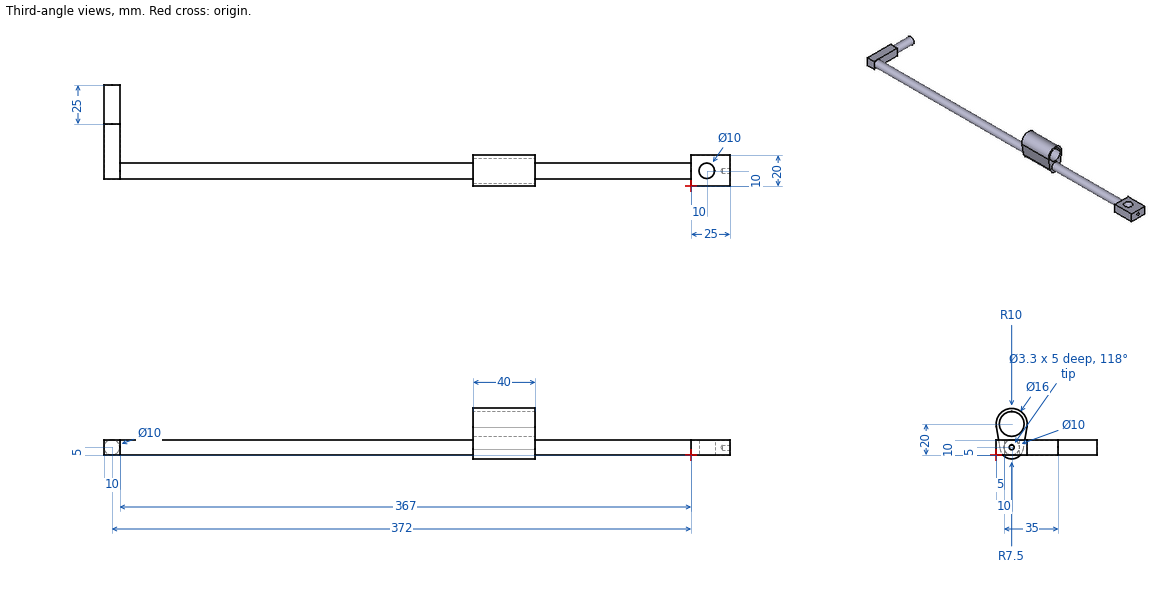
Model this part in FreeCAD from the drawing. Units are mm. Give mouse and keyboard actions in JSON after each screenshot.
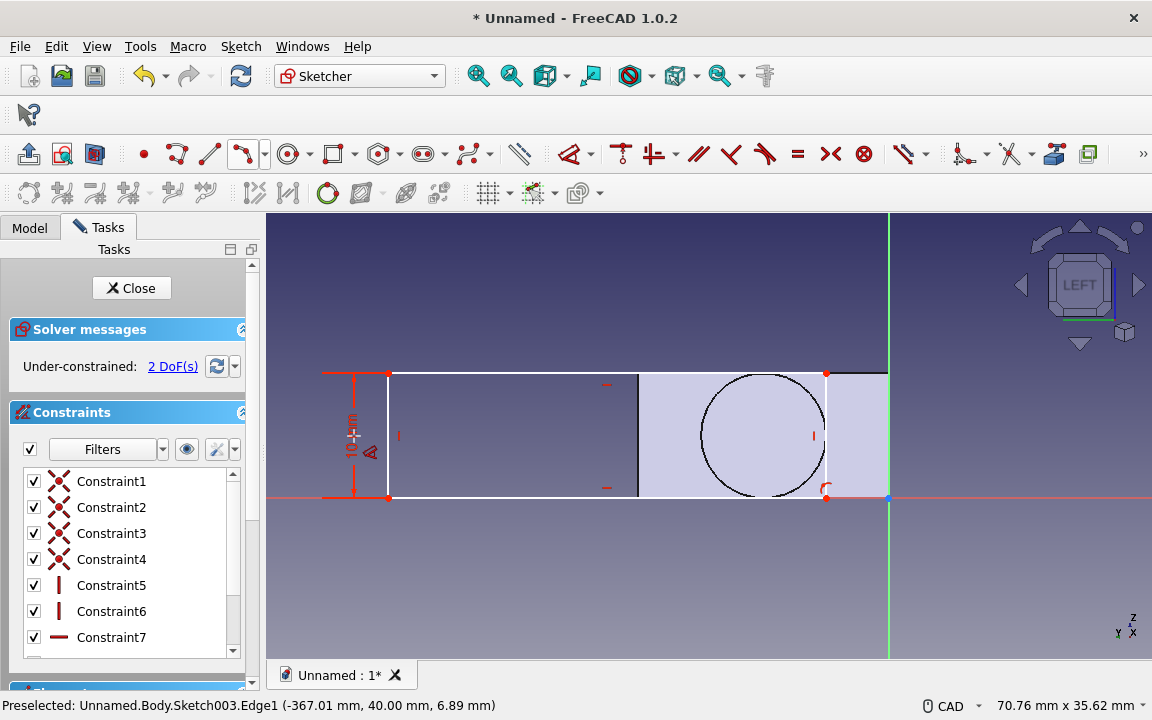
{"action": "left_click", "coordinate": [519, 498]}
{"action": "left_click", "coordinate": [607, 532]}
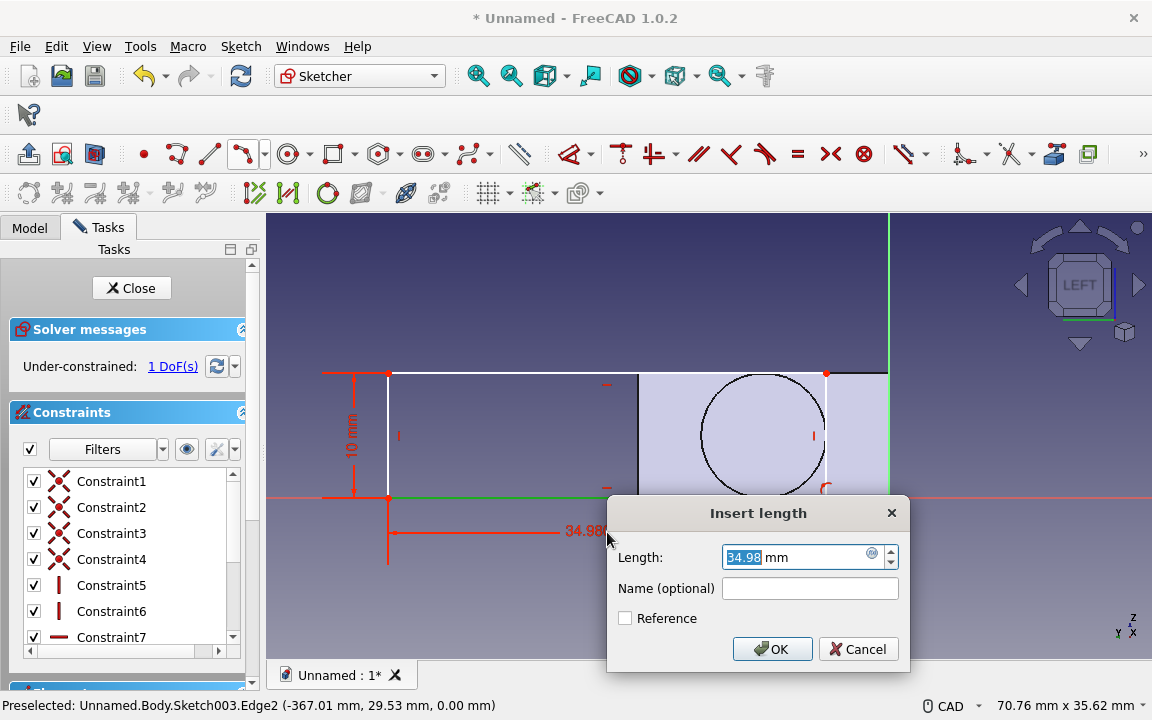
{"action": "type", "text": "35"}
{"action": "key", "text": "Return"}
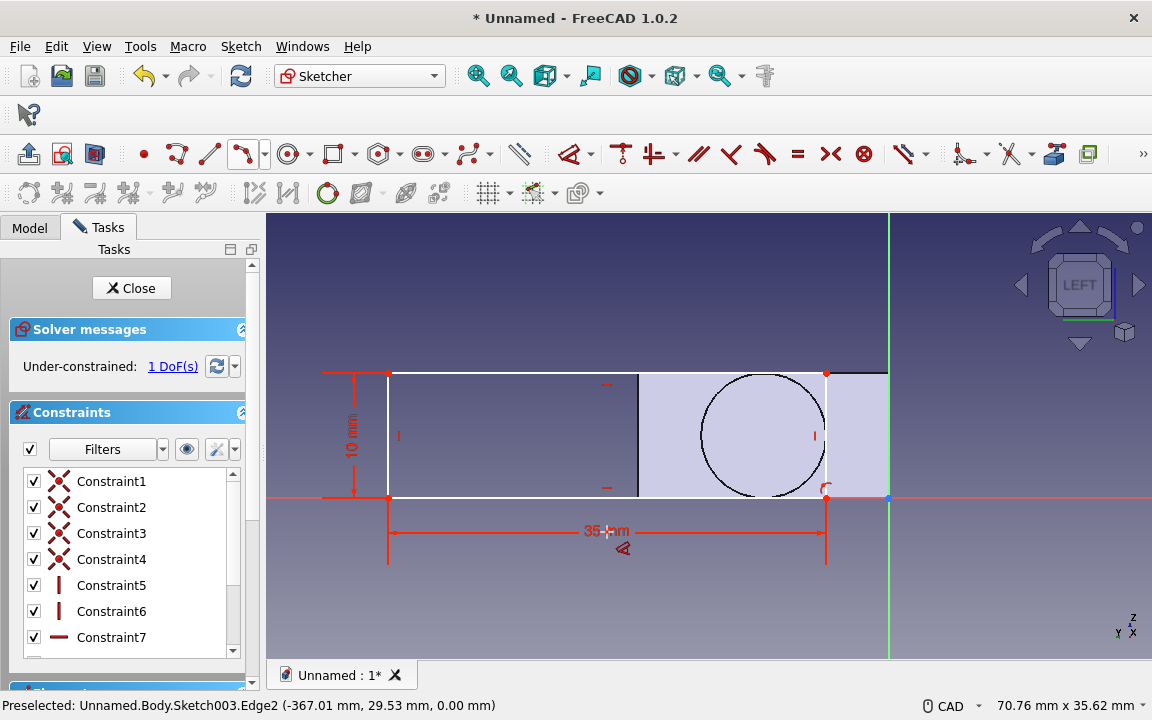
{"action": "left_click", "coordinate": [826, 498]}
{"action": "left_click", "coordinate": [858, 532]}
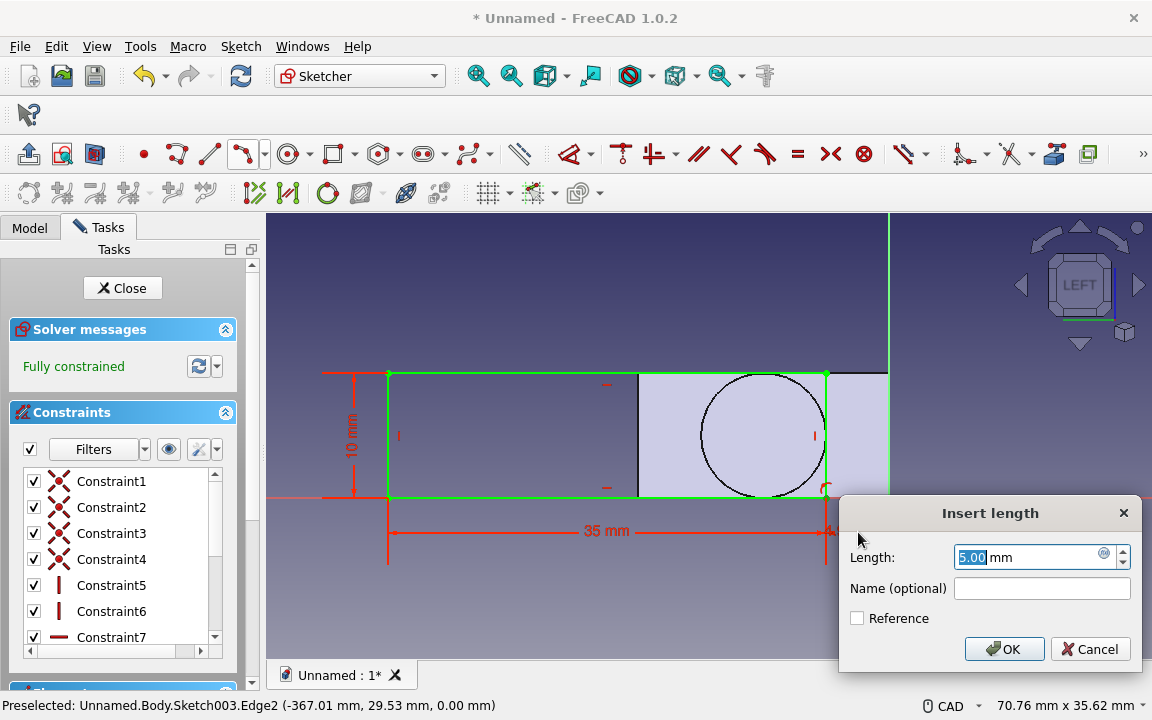
{"action": "type", "text": "5"}
{"action": "key", "text": "Return"}
{"action": "key", "text": "Escape"}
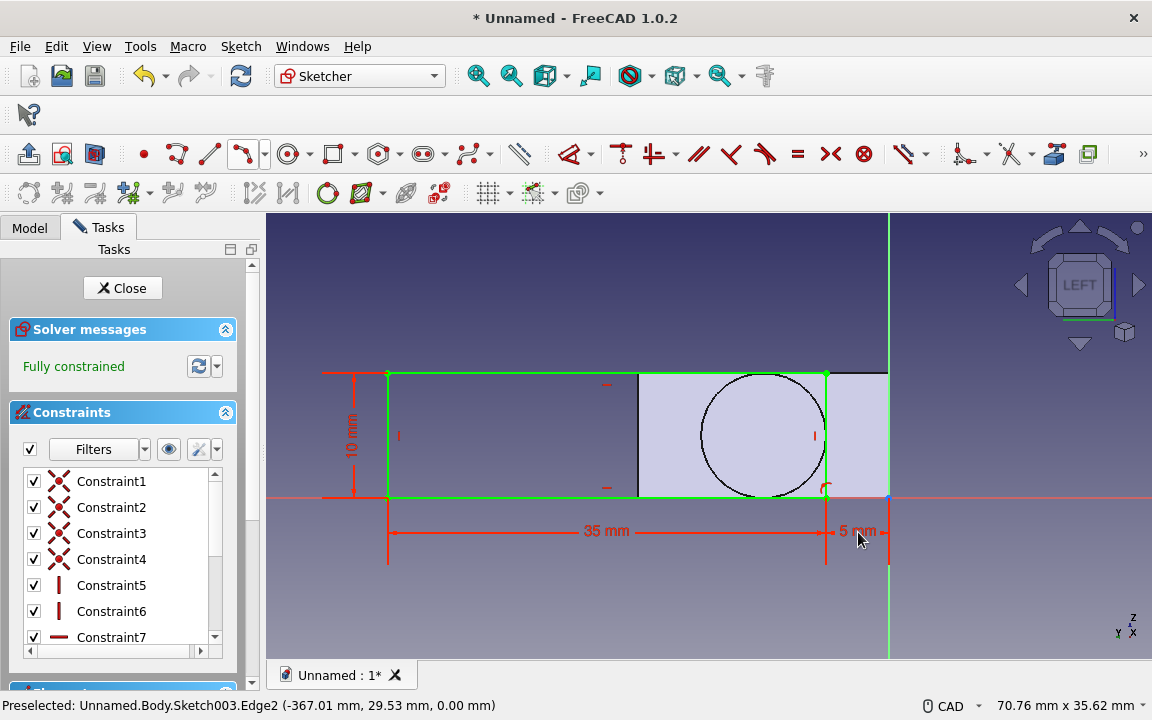
{"action": "left_click", "coordinate": [123, 288]}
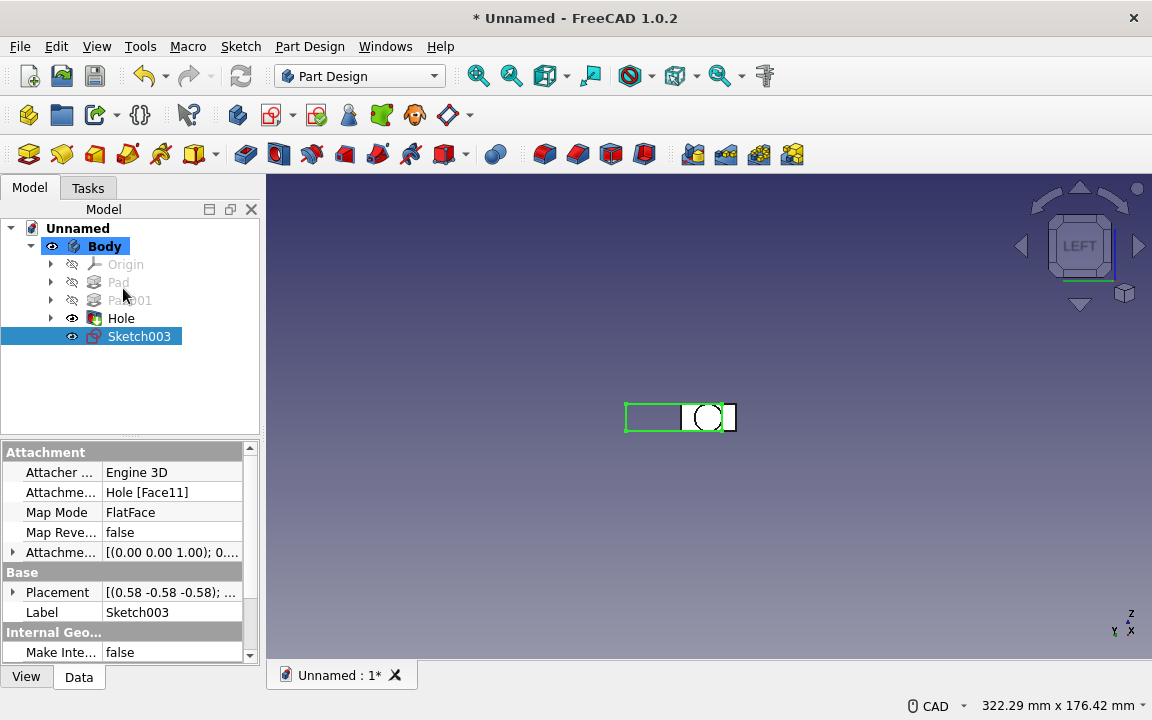
{"action": "left_click", "coordinate": [29, 154]}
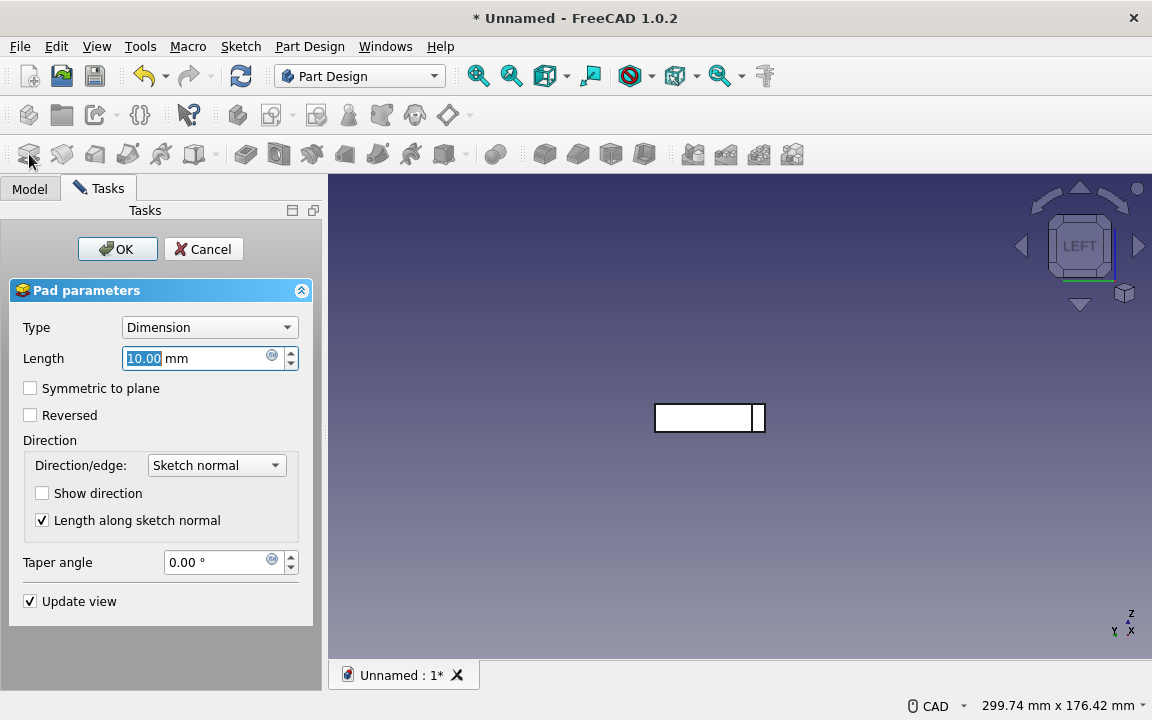
{"action": "type", "text": "10"}
{"action": "key", "text": "Tab"}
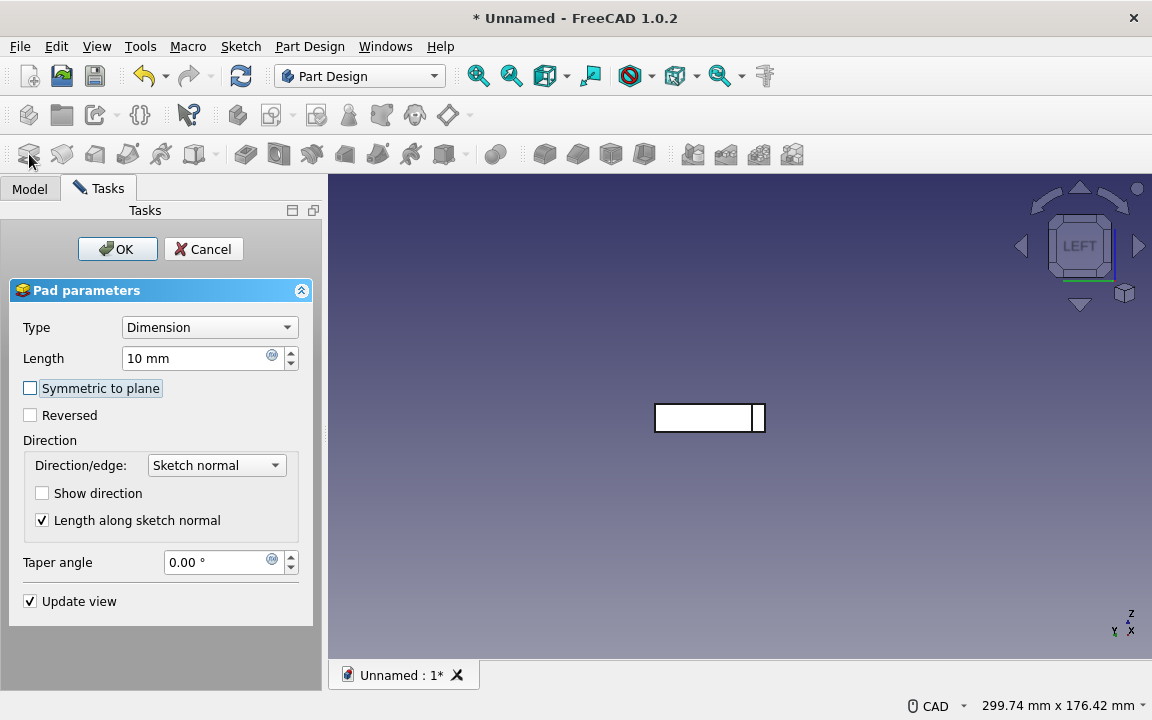
{"action": "left_click", "coordinate": [118, 249]}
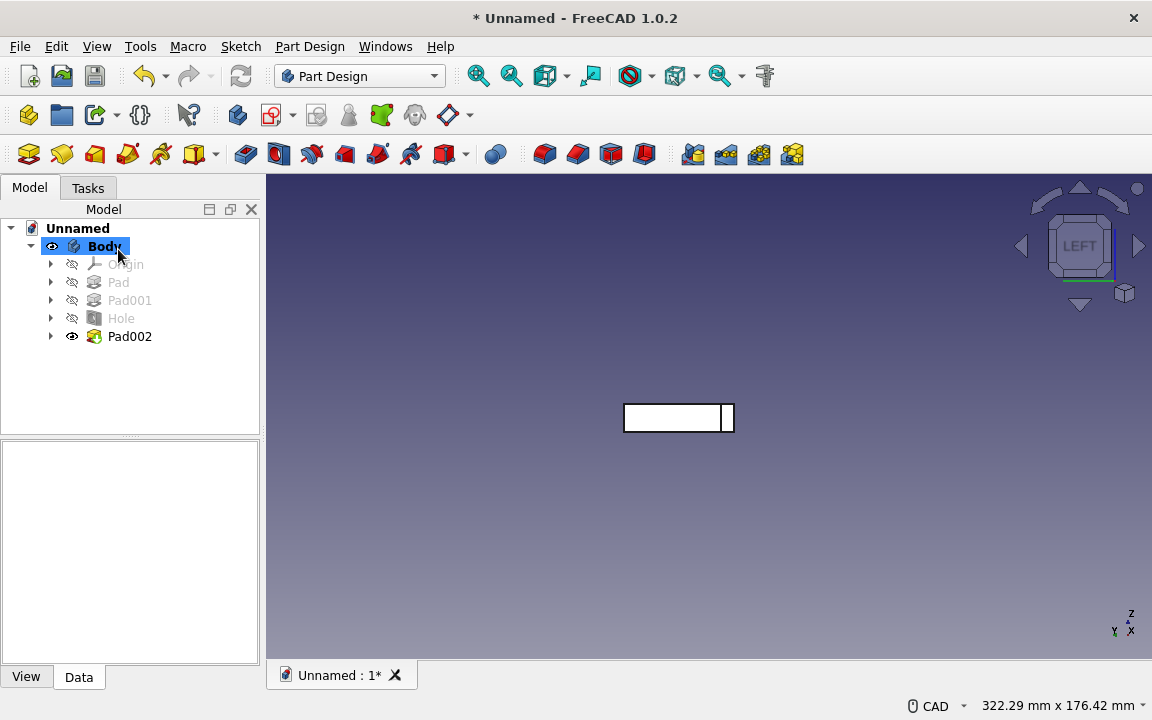
{"action": "key", "text": "v f"}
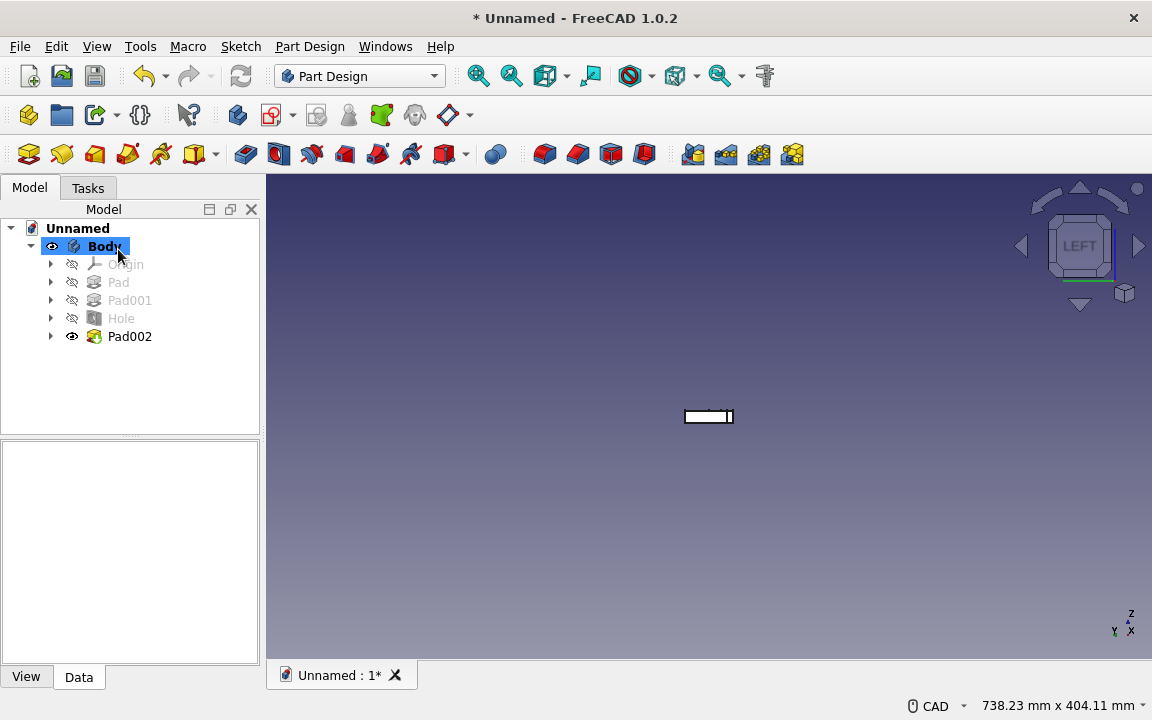
{"action": "key", "text": "4"}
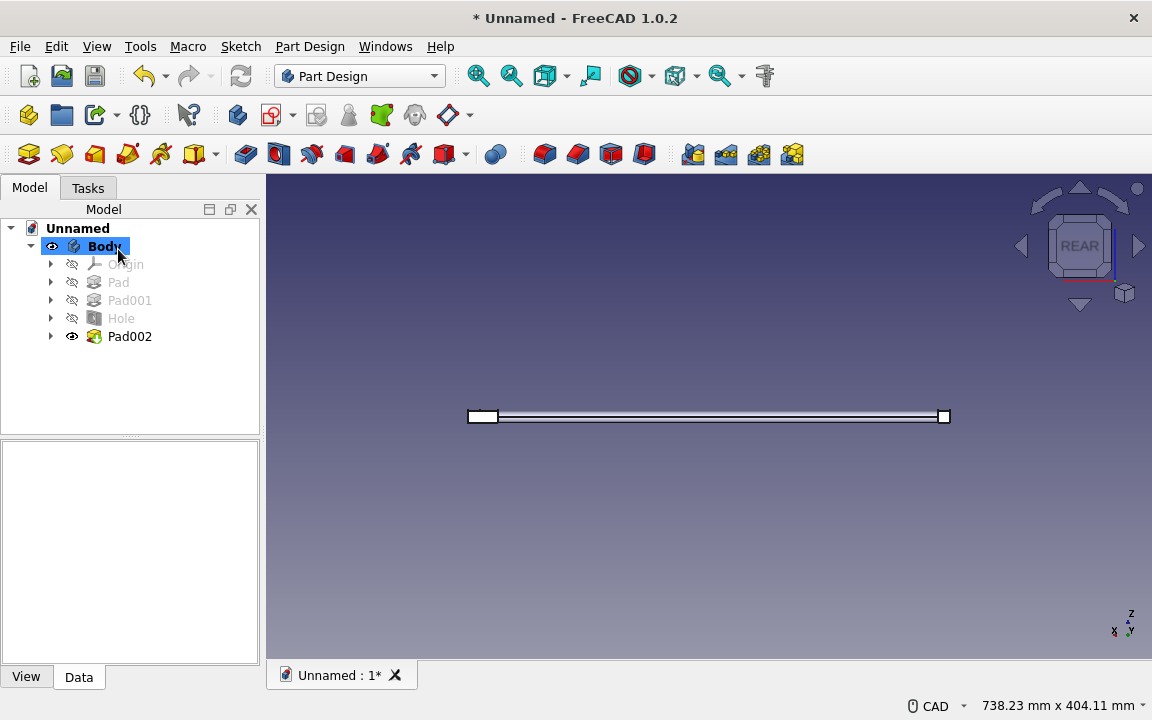
{"action": "scroll", "coordinate": [944, 415], "scroll_direction": "up", "scroll_amount": 4}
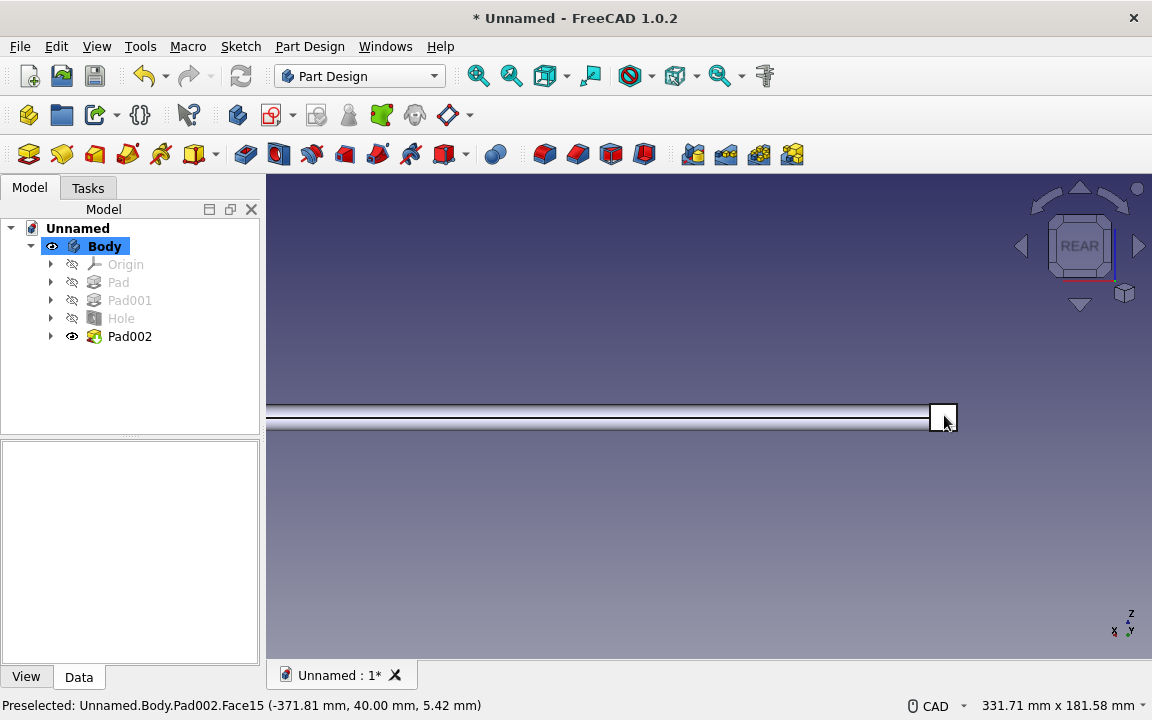
{"action": "left_click", "coordinate": [944, 417]}